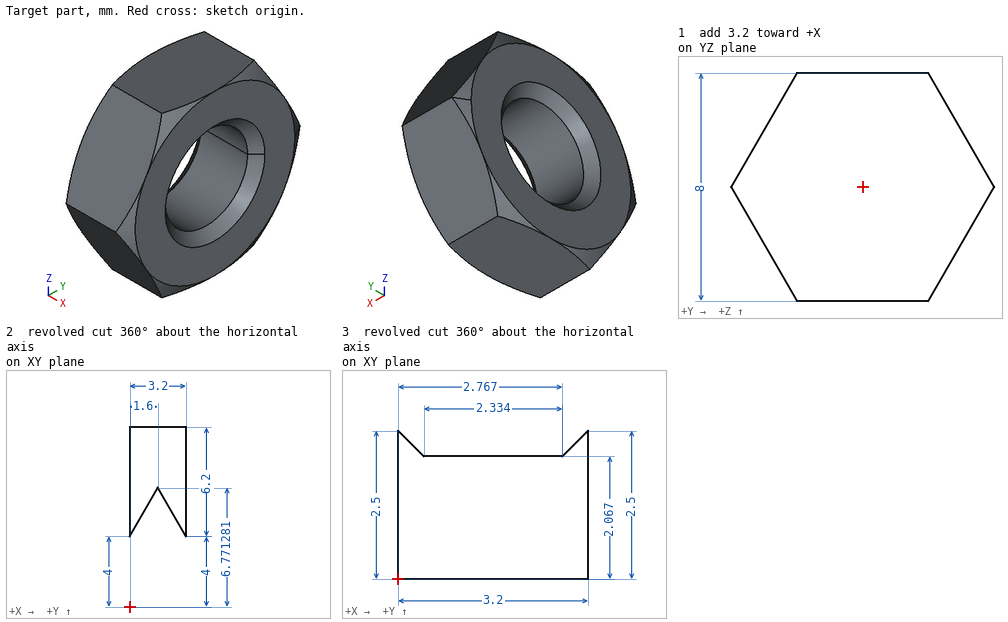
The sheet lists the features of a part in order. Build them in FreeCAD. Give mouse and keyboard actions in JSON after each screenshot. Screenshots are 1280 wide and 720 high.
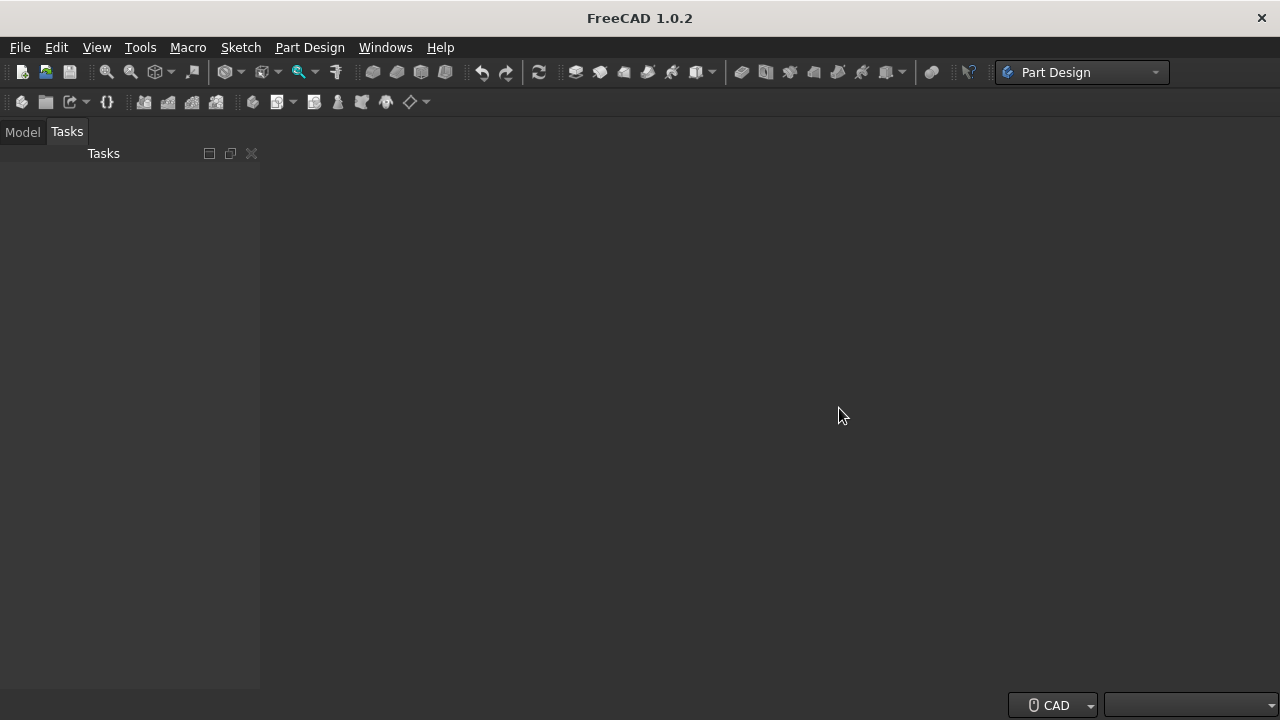
{"action": "key", "text": "ctrl+n"}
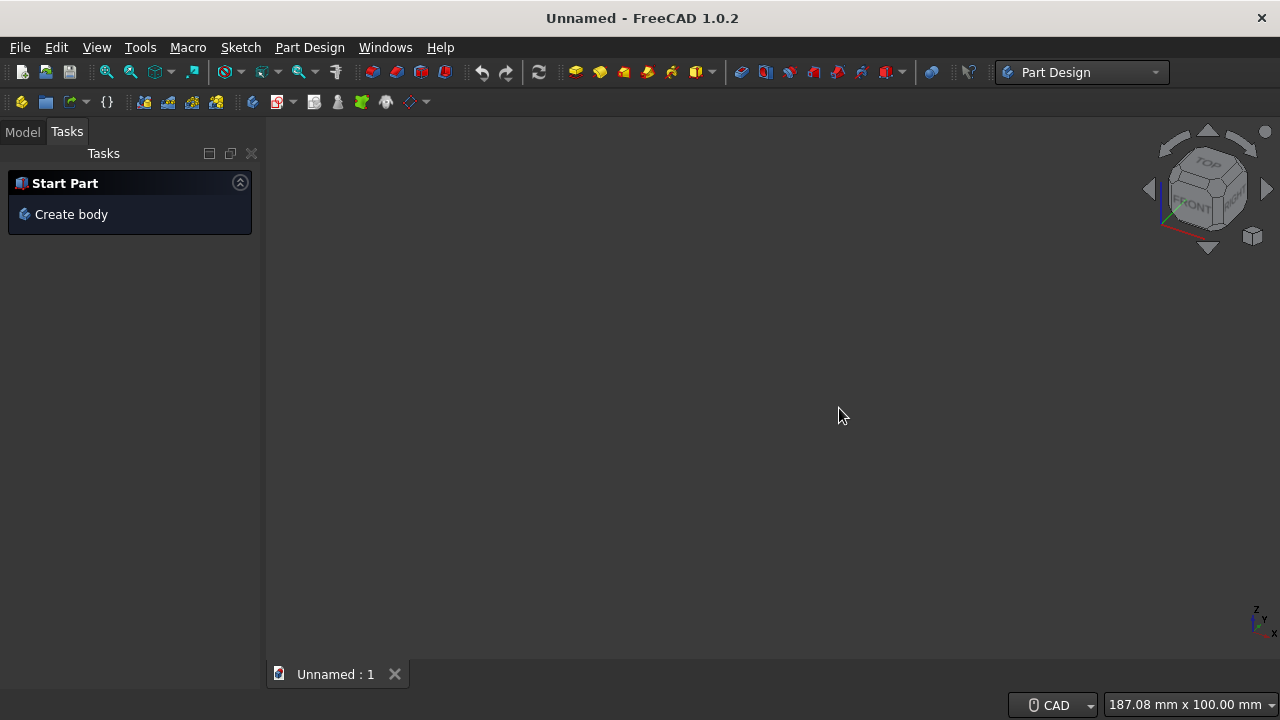
{"action": "left_click", "coordinate": [278, 102]}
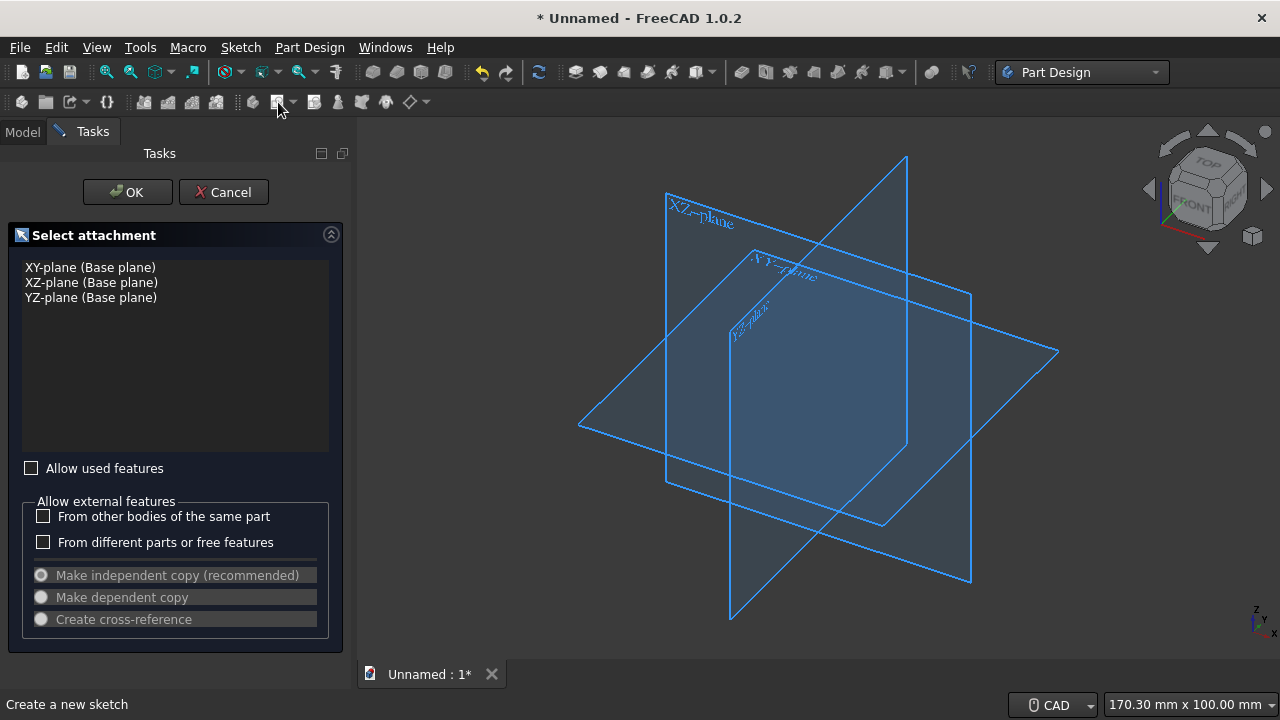
{"action": "left_click", "coordinate": [82, 298]}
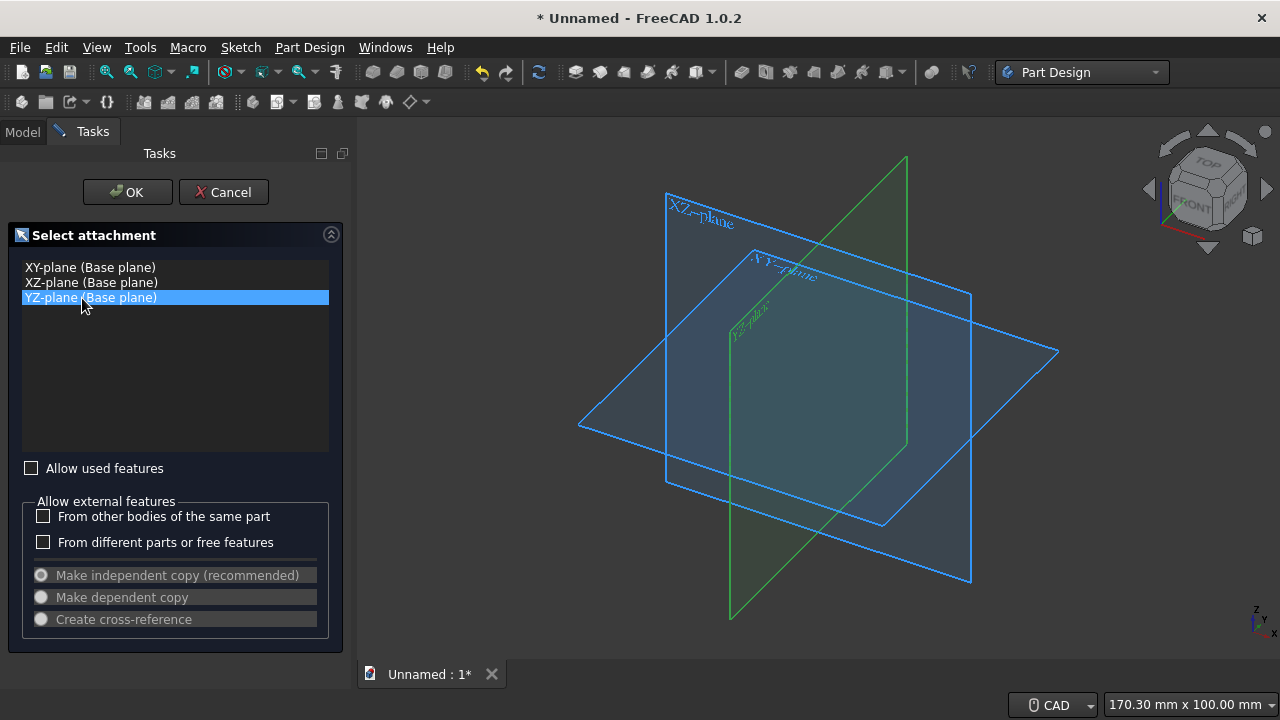
{"action": "left_click", "coordinate": [128, 192]}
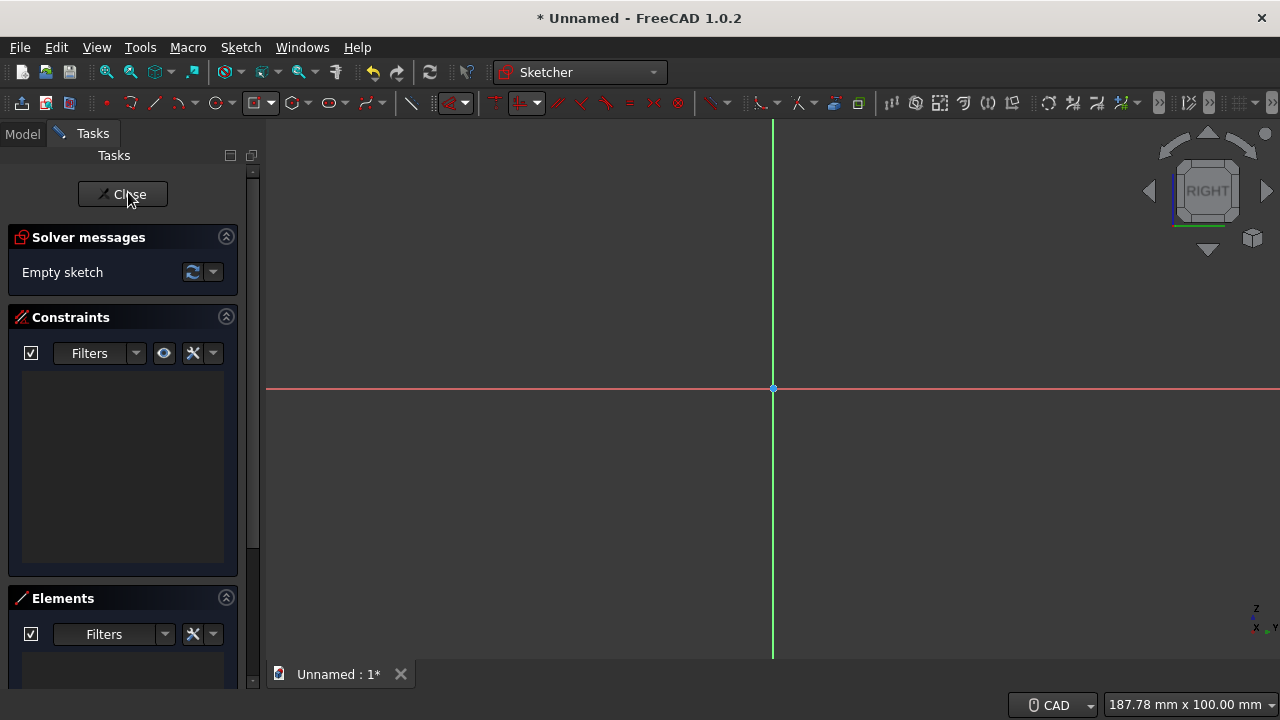
{"action": "scroll", "coordinate": [784, 389], "scroll_direction": "up", "scroll_amount": 10}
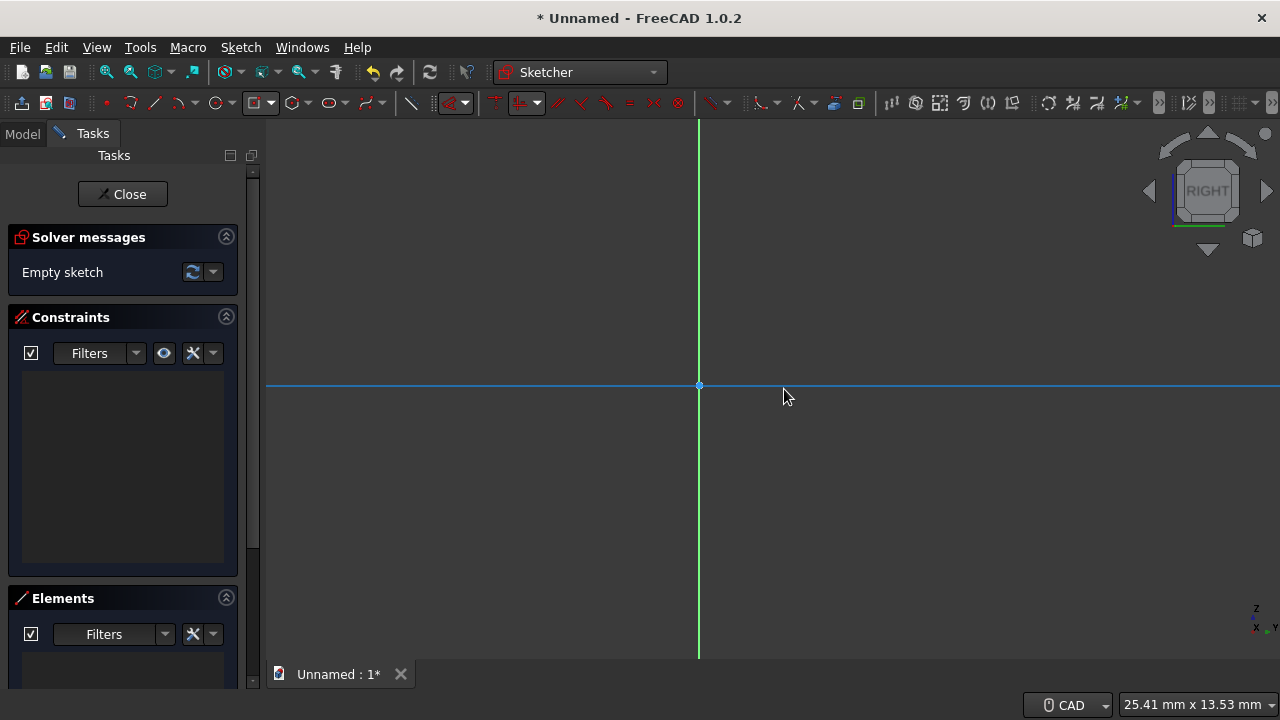
{"action": "key", "text": "g p 6"}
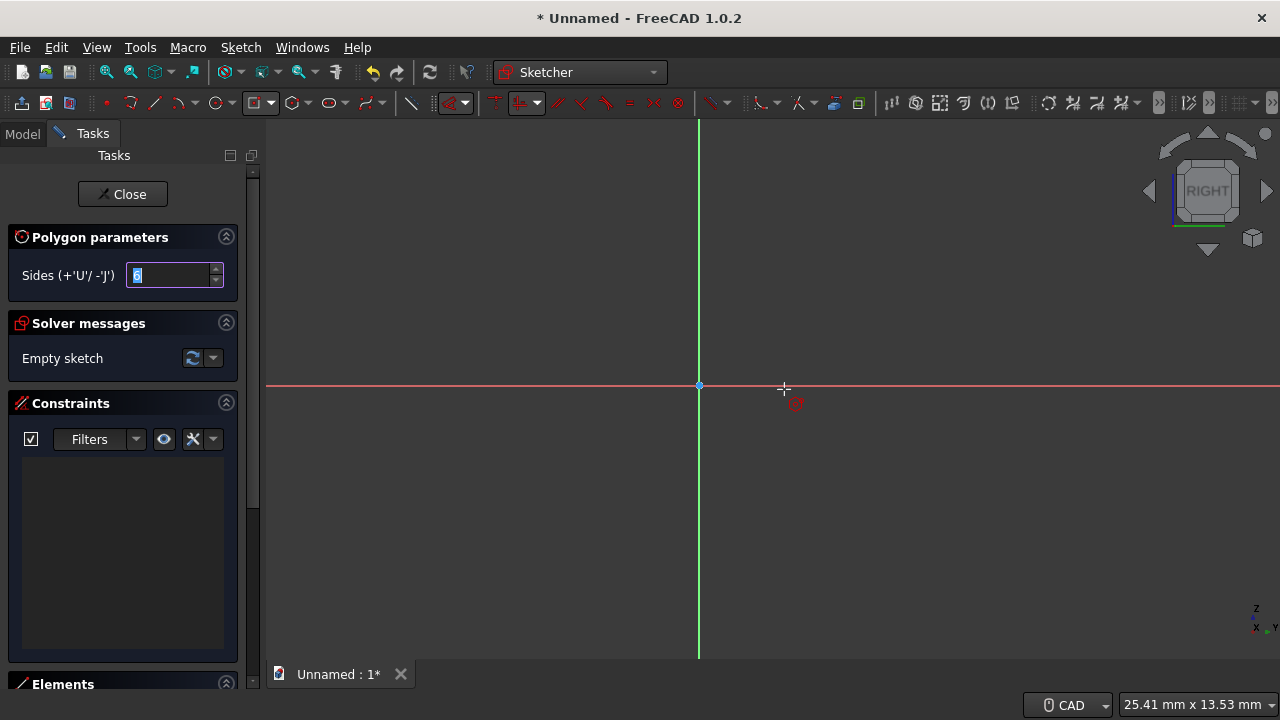
{"action": "left_click", "coordinate": [699, 386]}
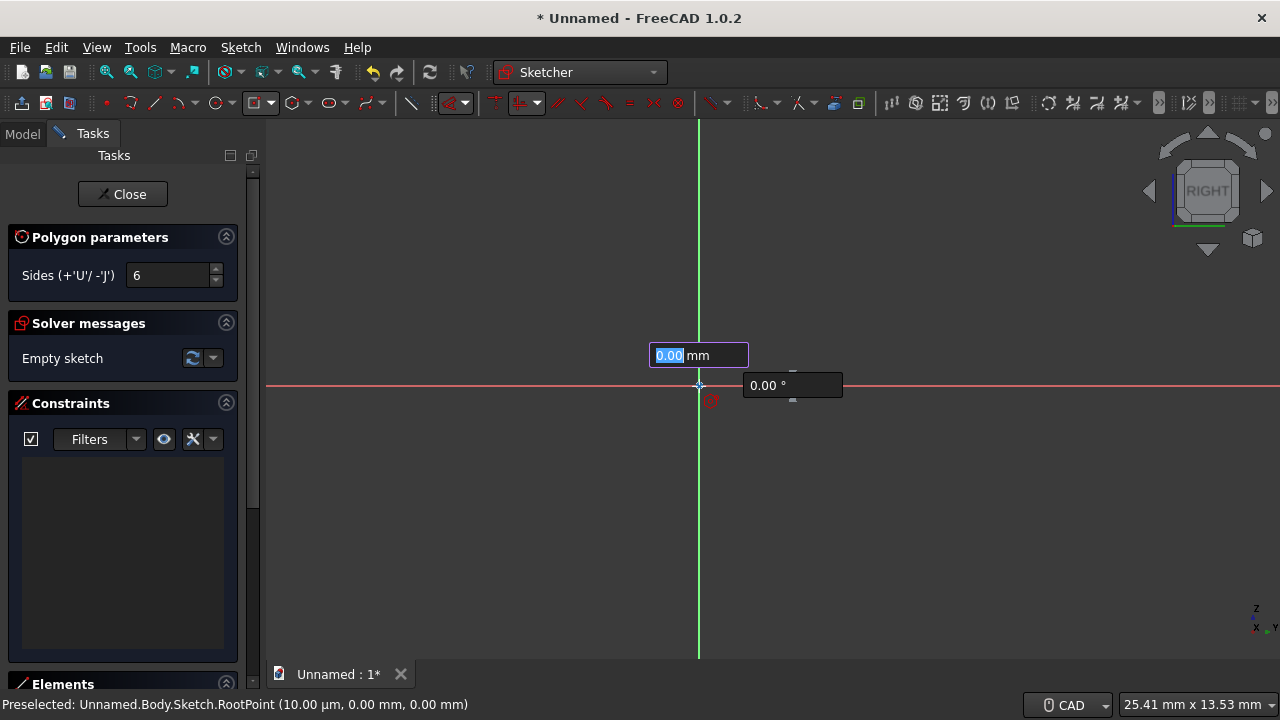
{"action": "left_click", "coordinate": [515, 386]}
{"action": "right_click", "coordinate": [515, 386]}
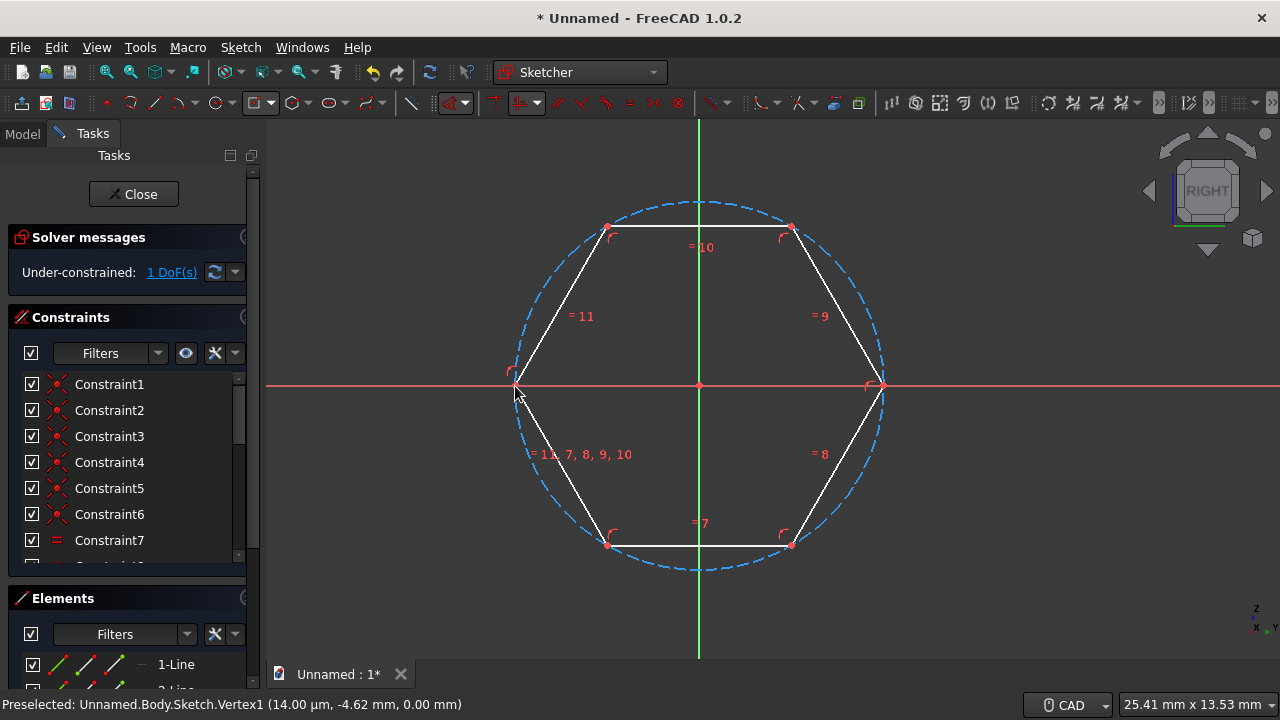
{"action": "key", "text": "d"}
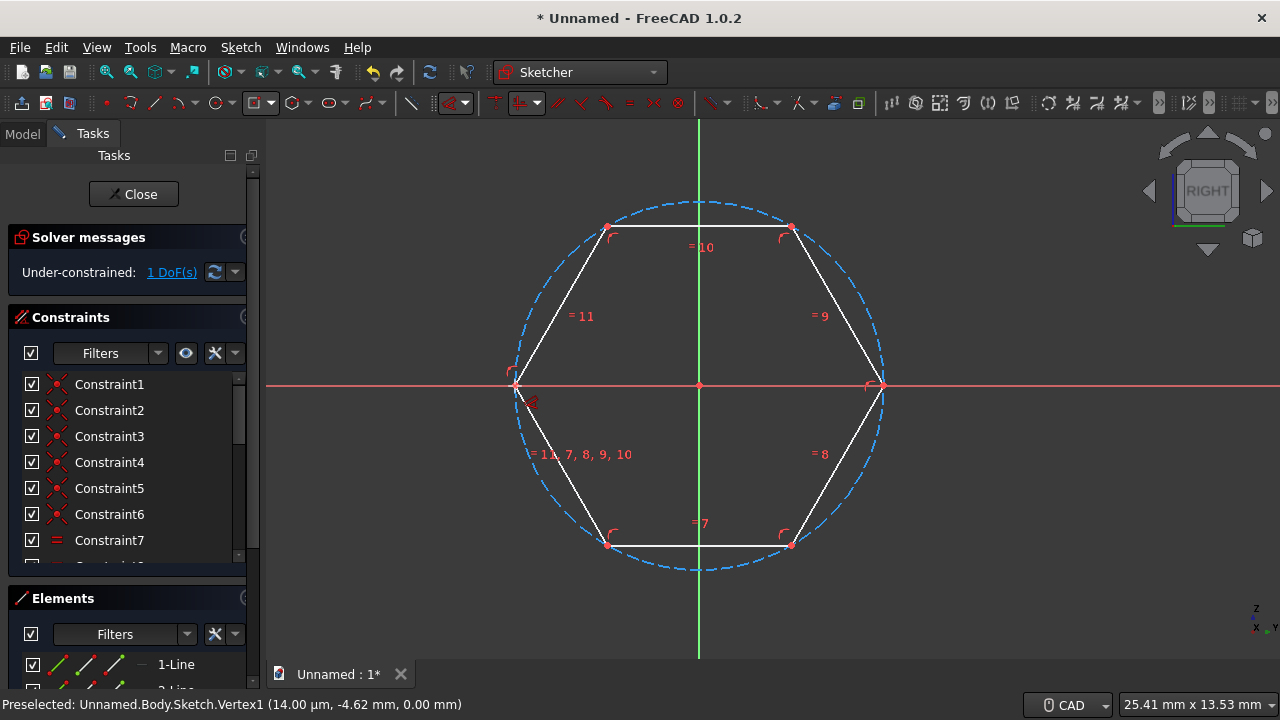
{"action": "left_click", "coordinate": [607, 546]}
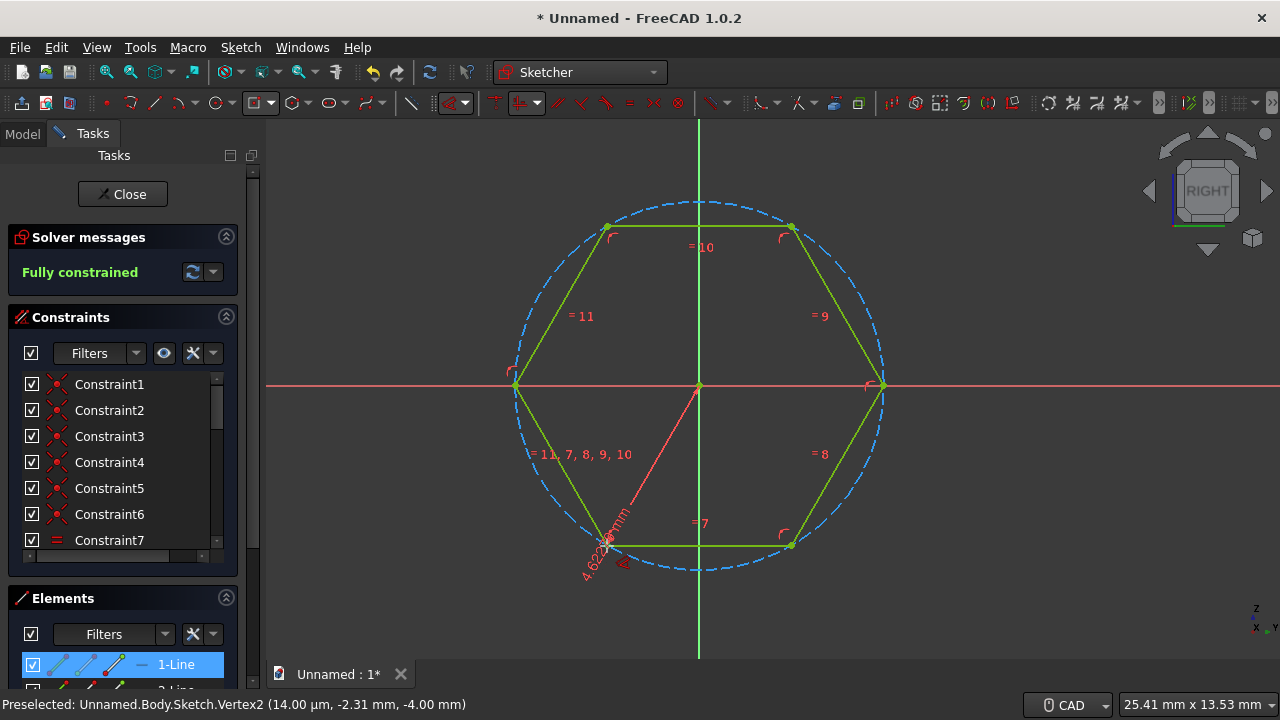
{"action": "left_click", "coordinate": [792, 226]}
{"action": "left_click", "coordinate": [826, 312]}